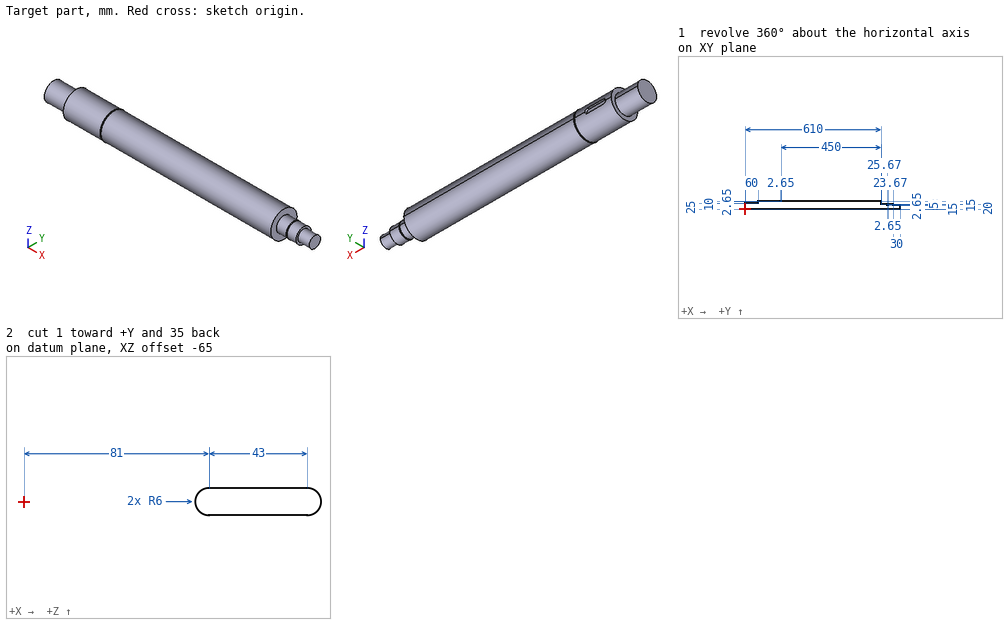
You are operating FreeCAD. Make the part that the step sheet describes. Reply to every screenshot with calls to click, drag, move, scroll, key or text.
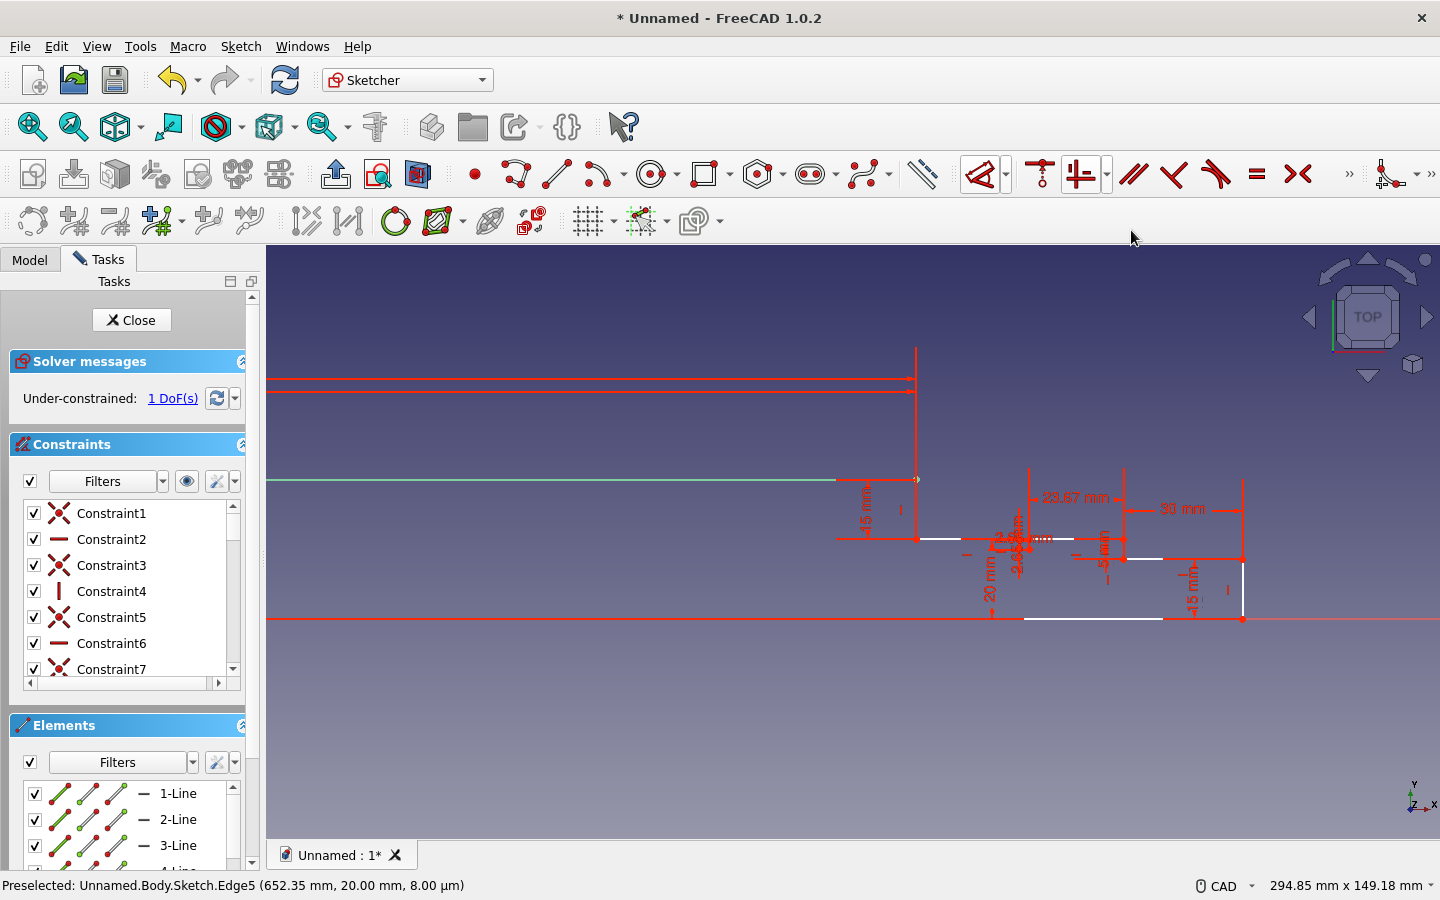
click(988, 539)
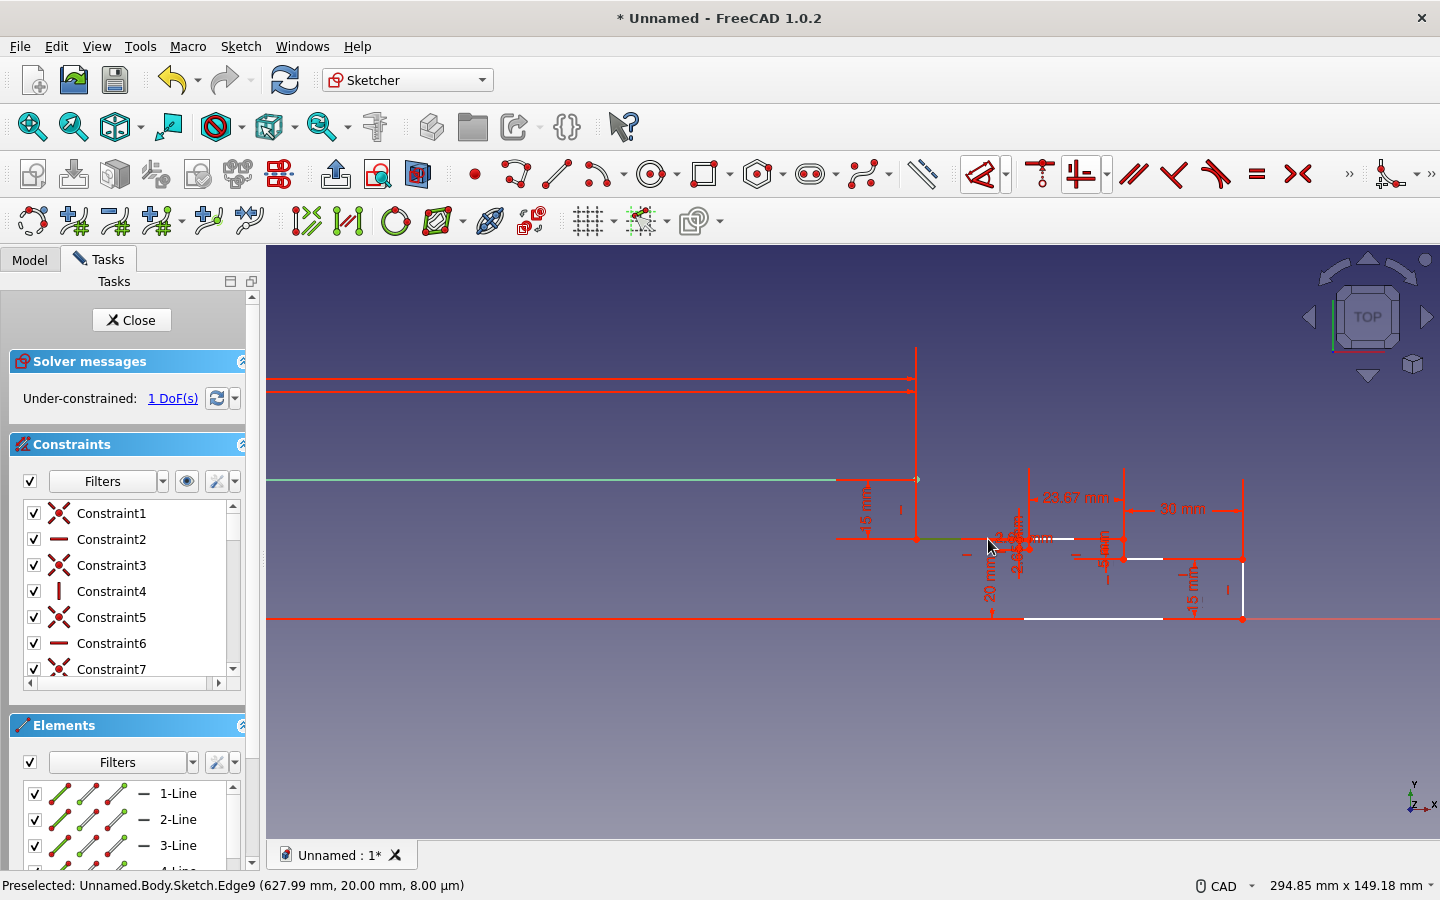
click(1006, 174)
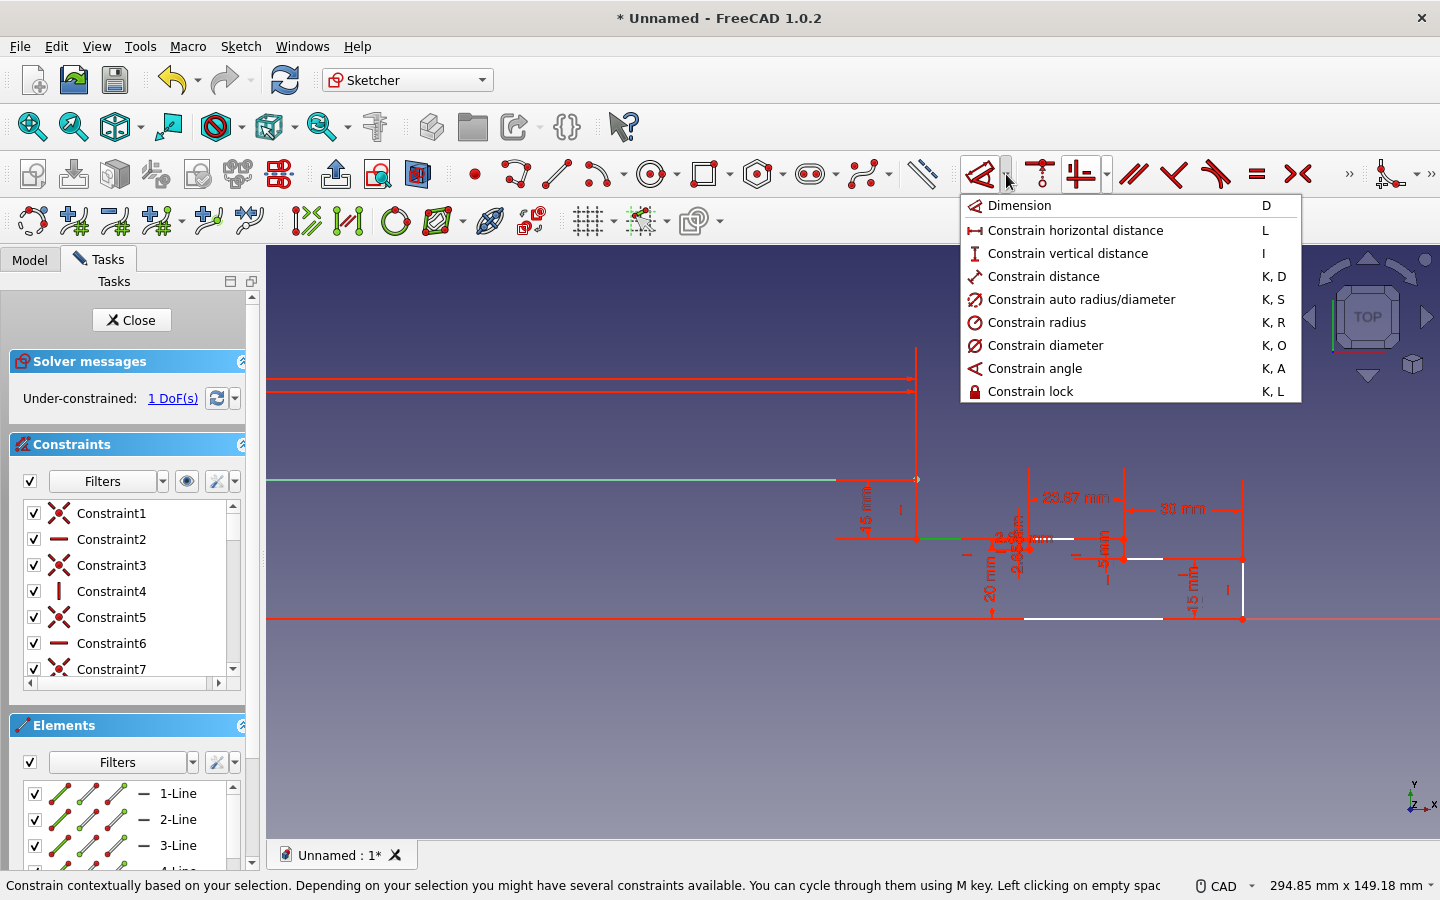
click(1131, 230)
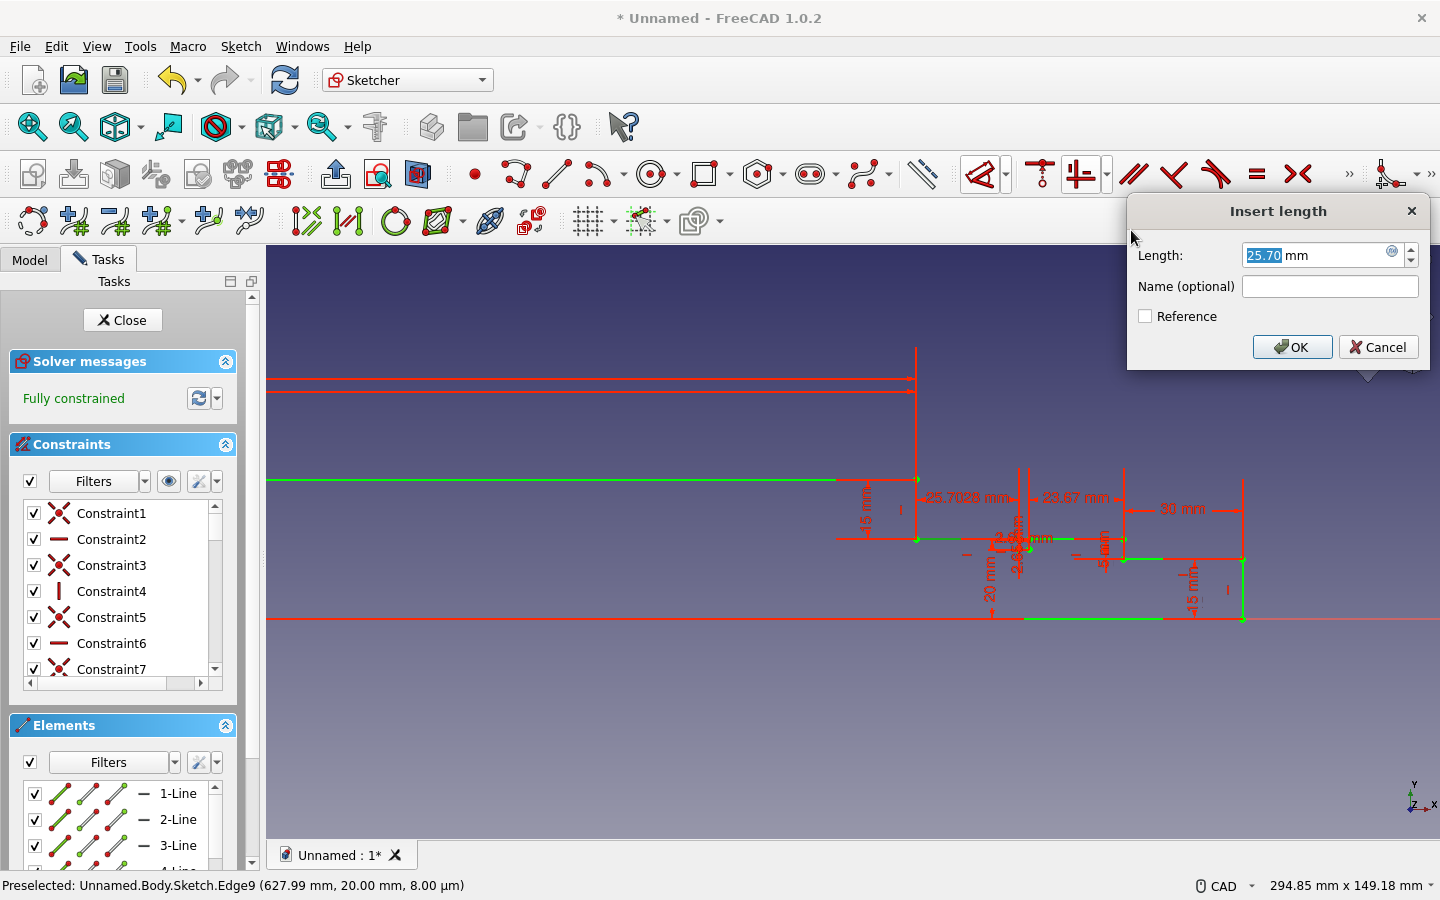
text(25.67)
key(Return)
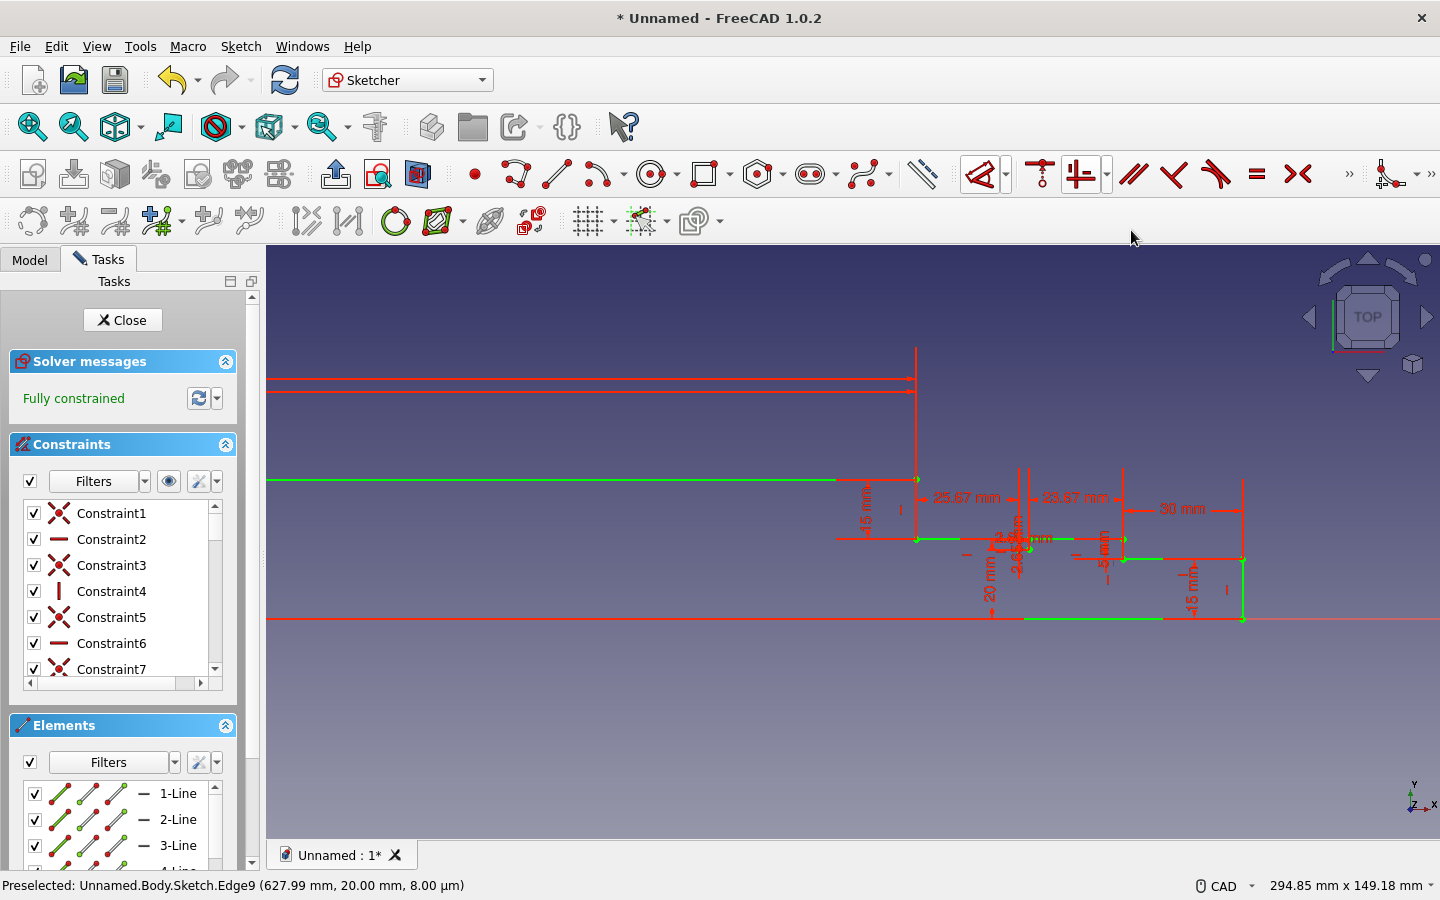
click(123, 320)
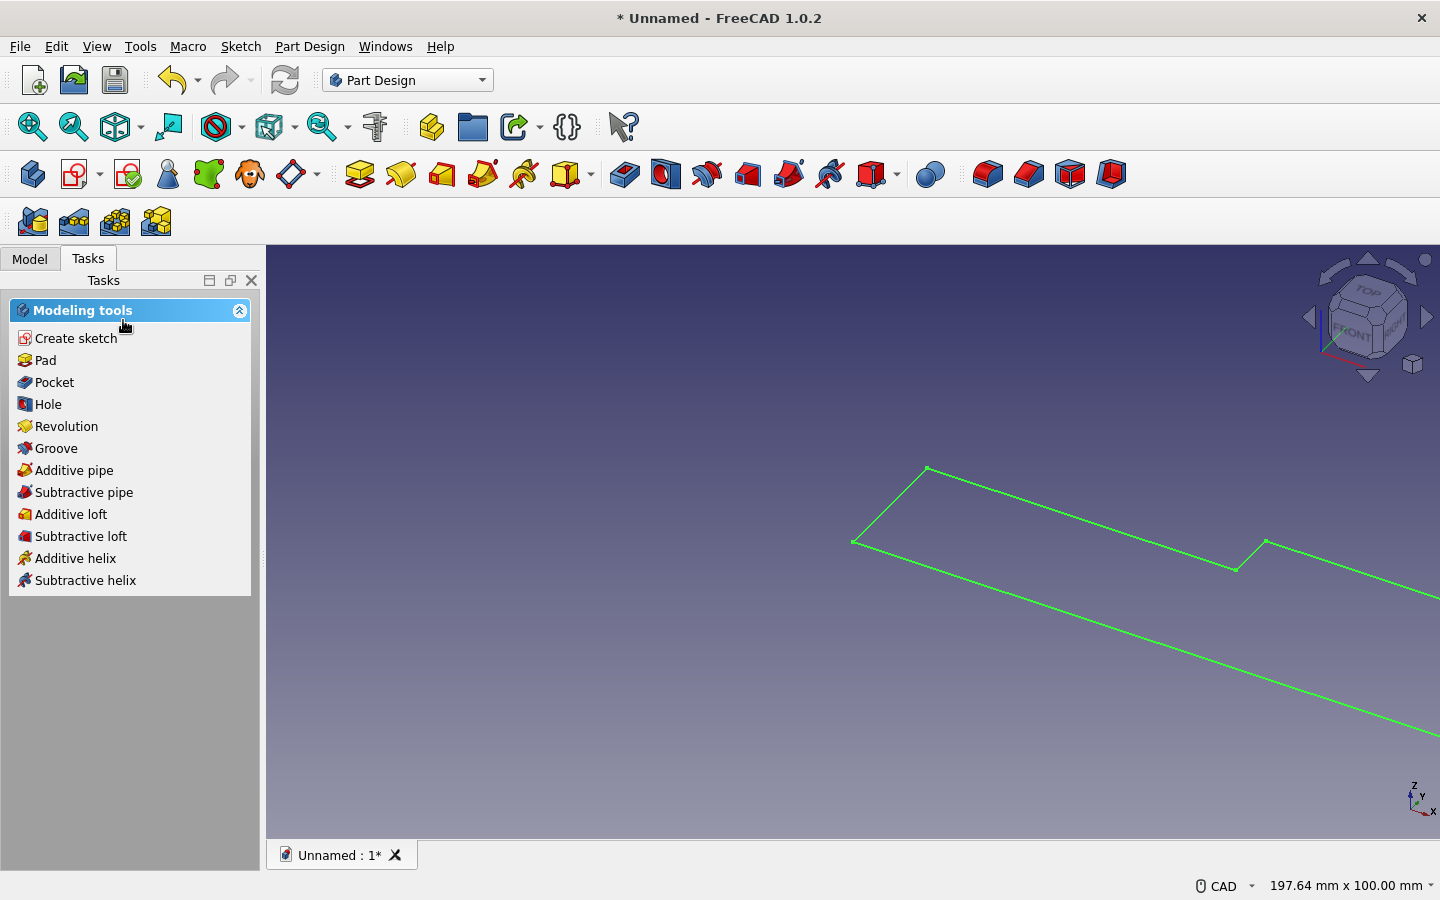
click(401, 174)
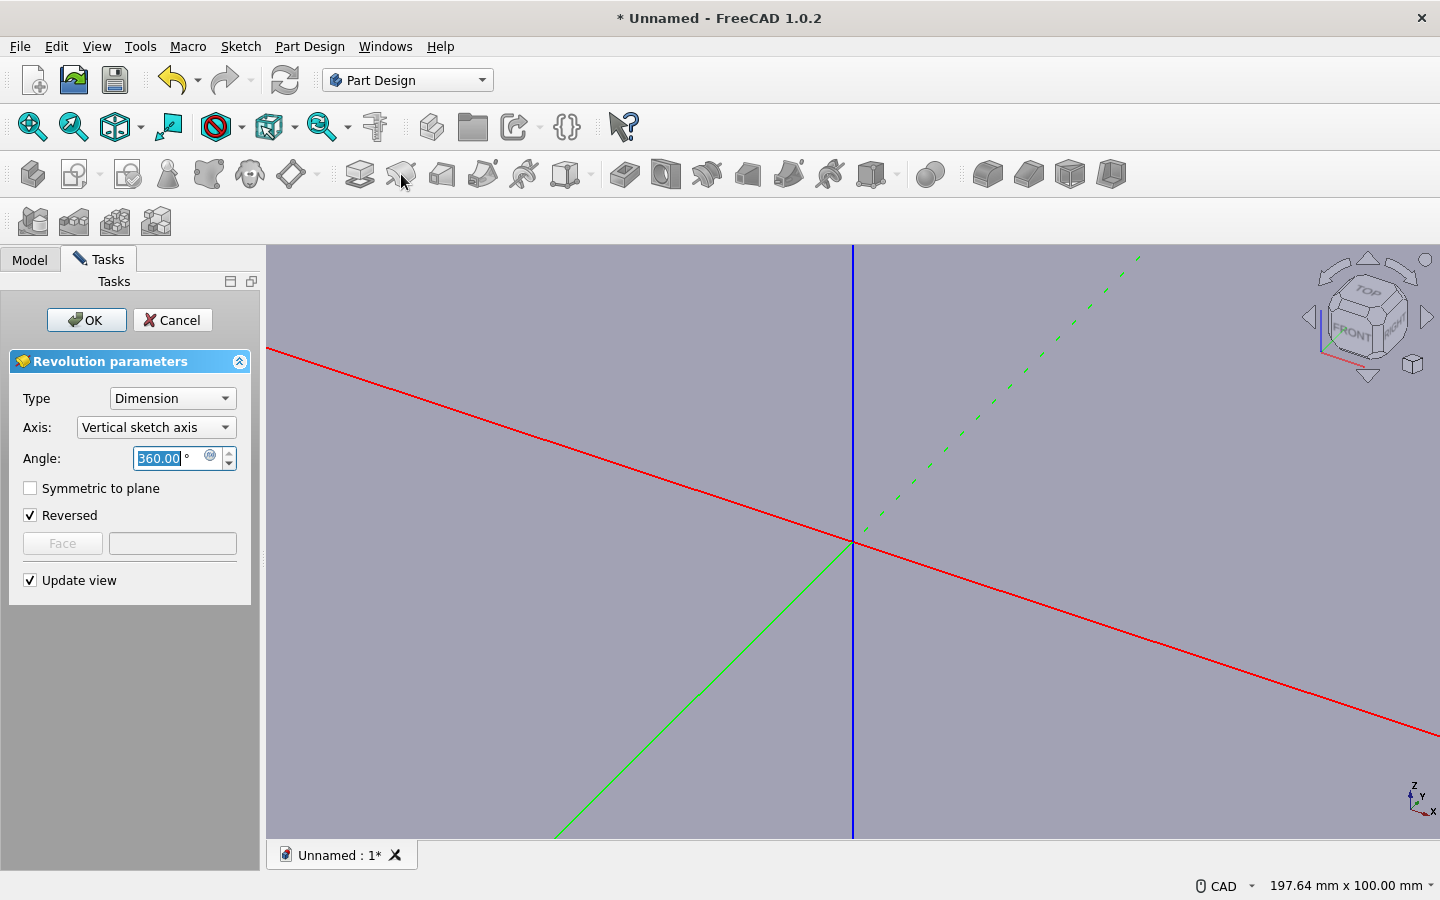
click(157, 428)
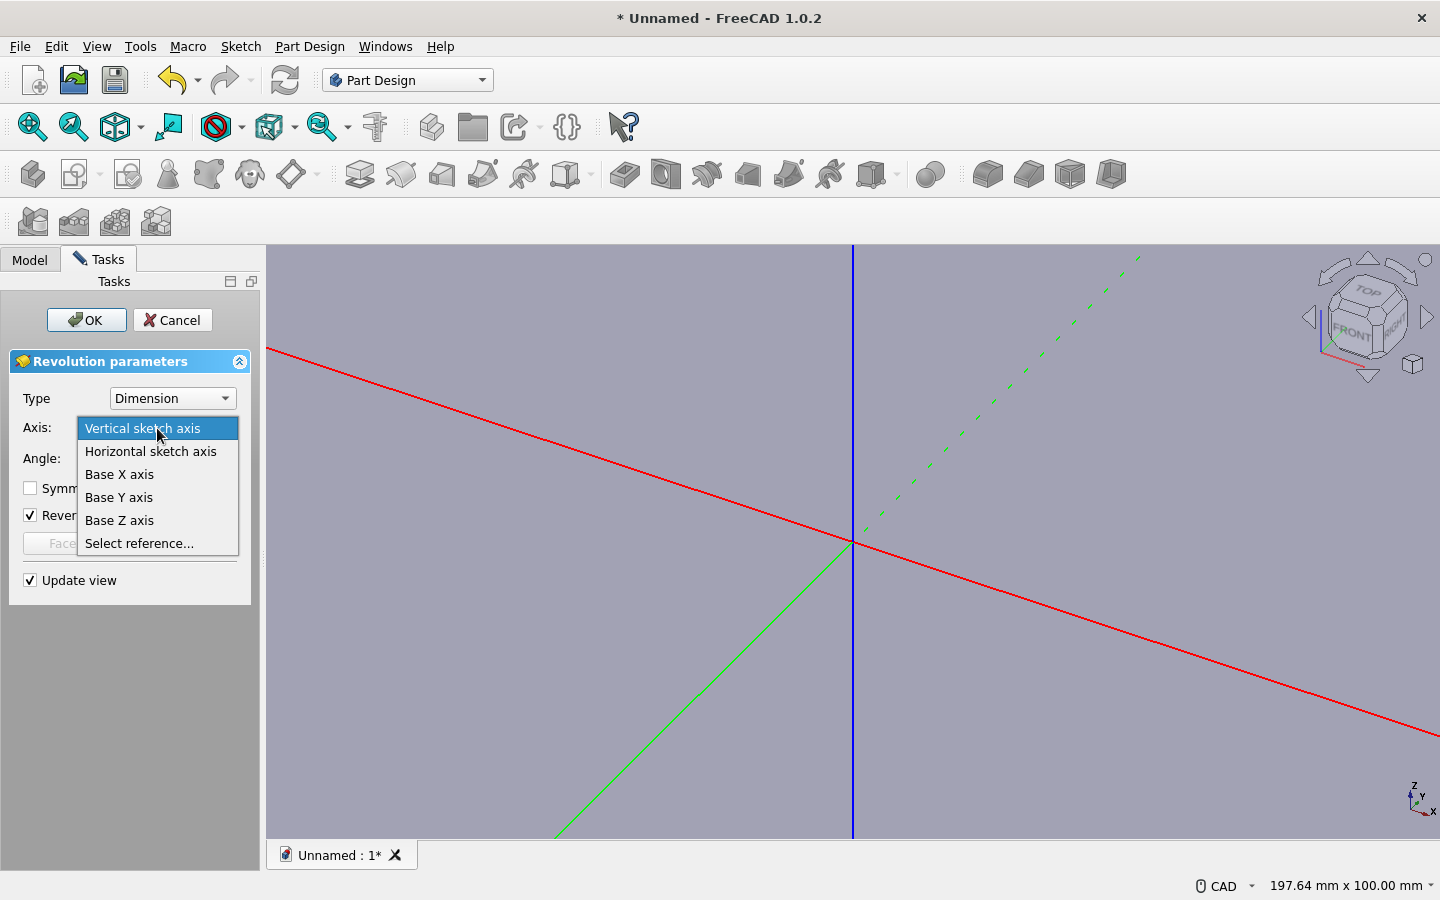
click(156, 452)